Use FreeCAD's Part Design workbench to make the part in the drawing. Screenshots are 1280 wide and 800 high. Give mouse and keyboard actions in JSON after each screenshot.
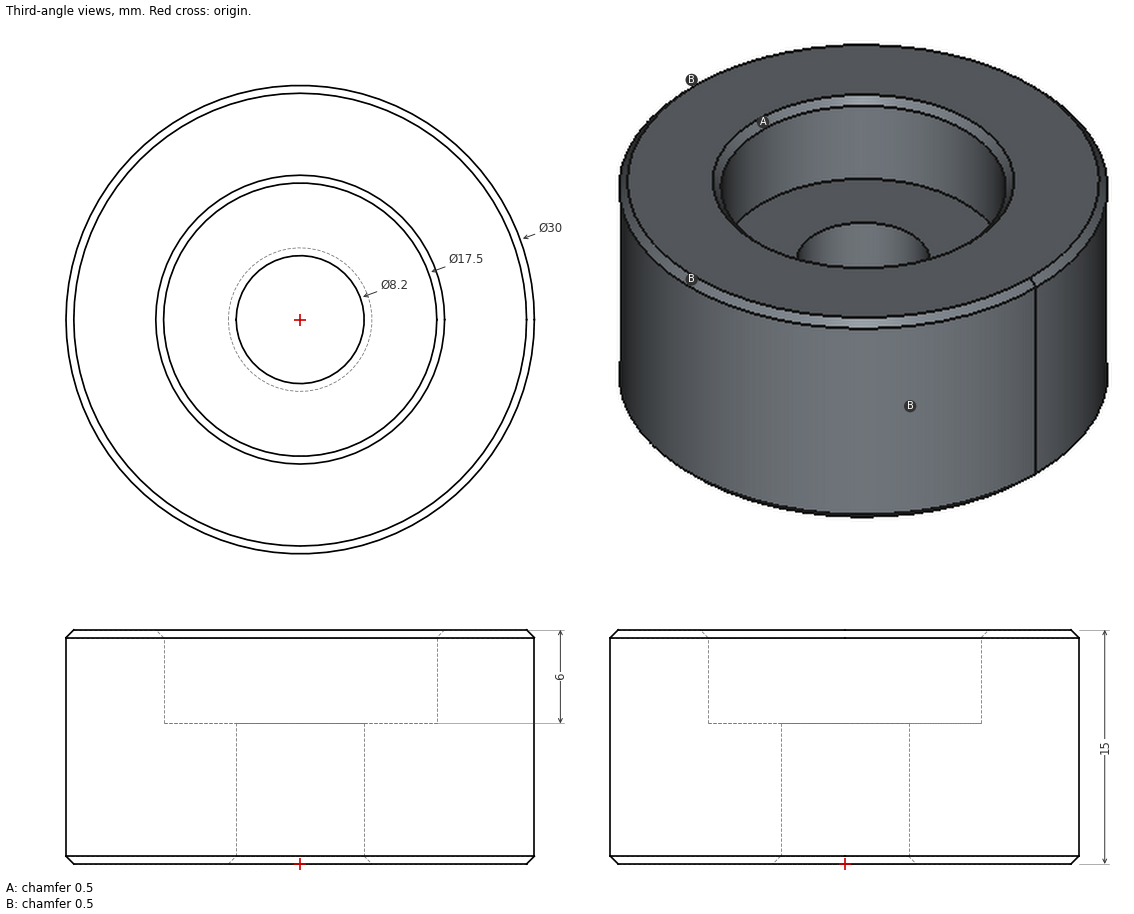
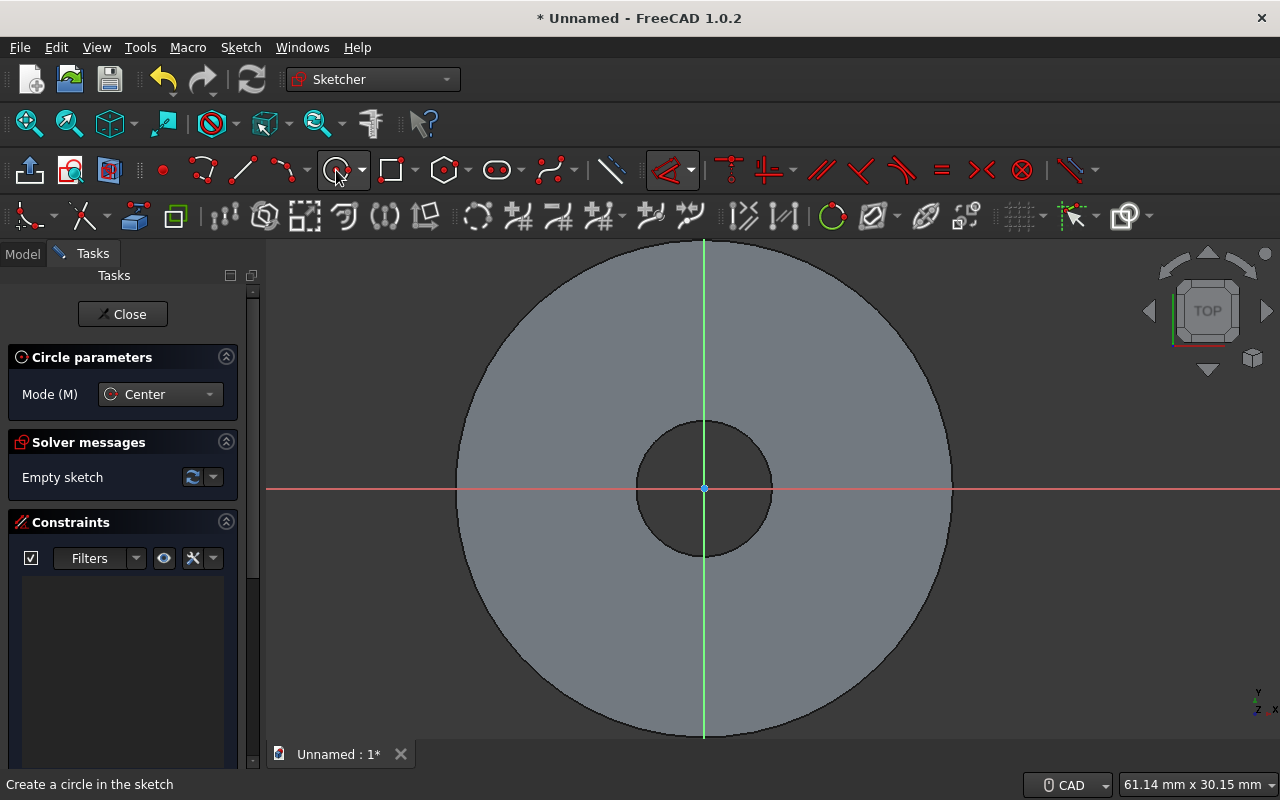
{"action": "left_click", "coordinate": [704, 489]}
{"action": "mouse_move", "coordinate": [807, 386]}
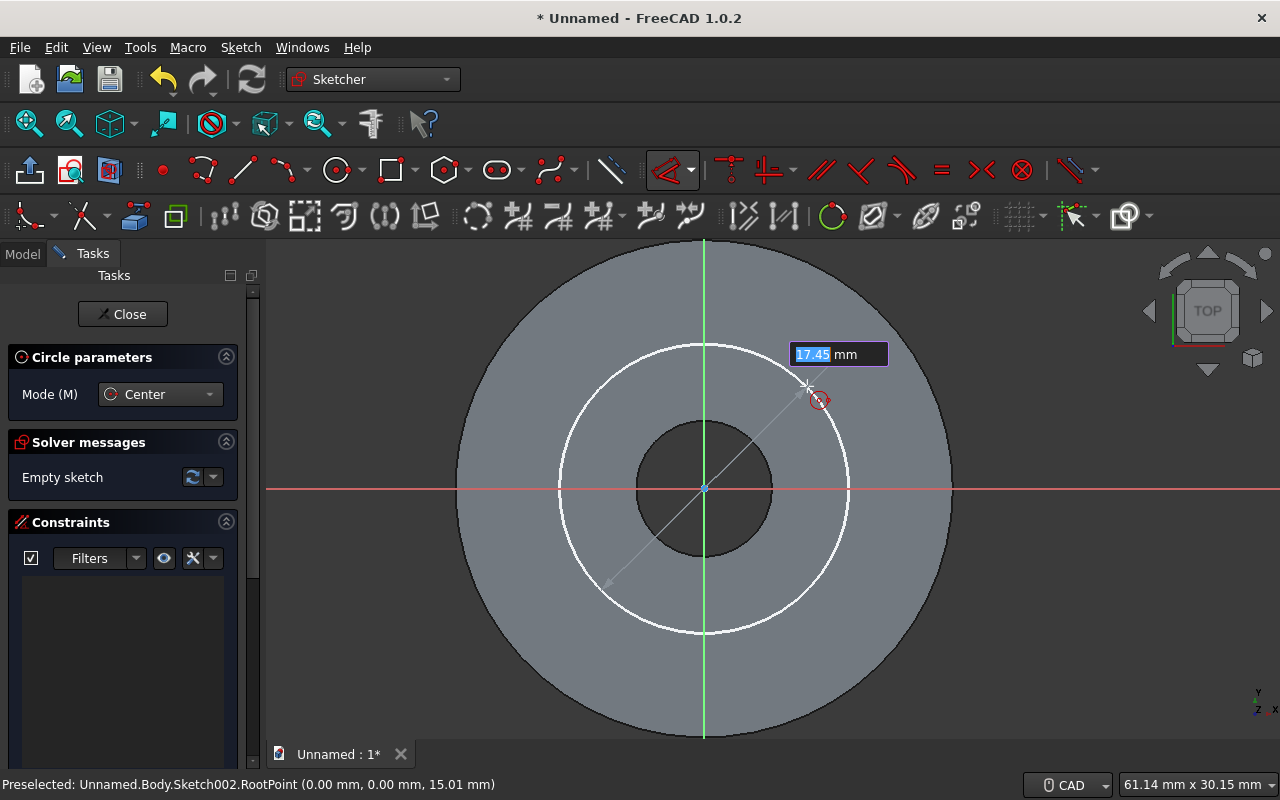
{"action": "type", "text": "17.5"}
{"action": "key", "text": "Return"}
{"action": "key", "text": "Escape"}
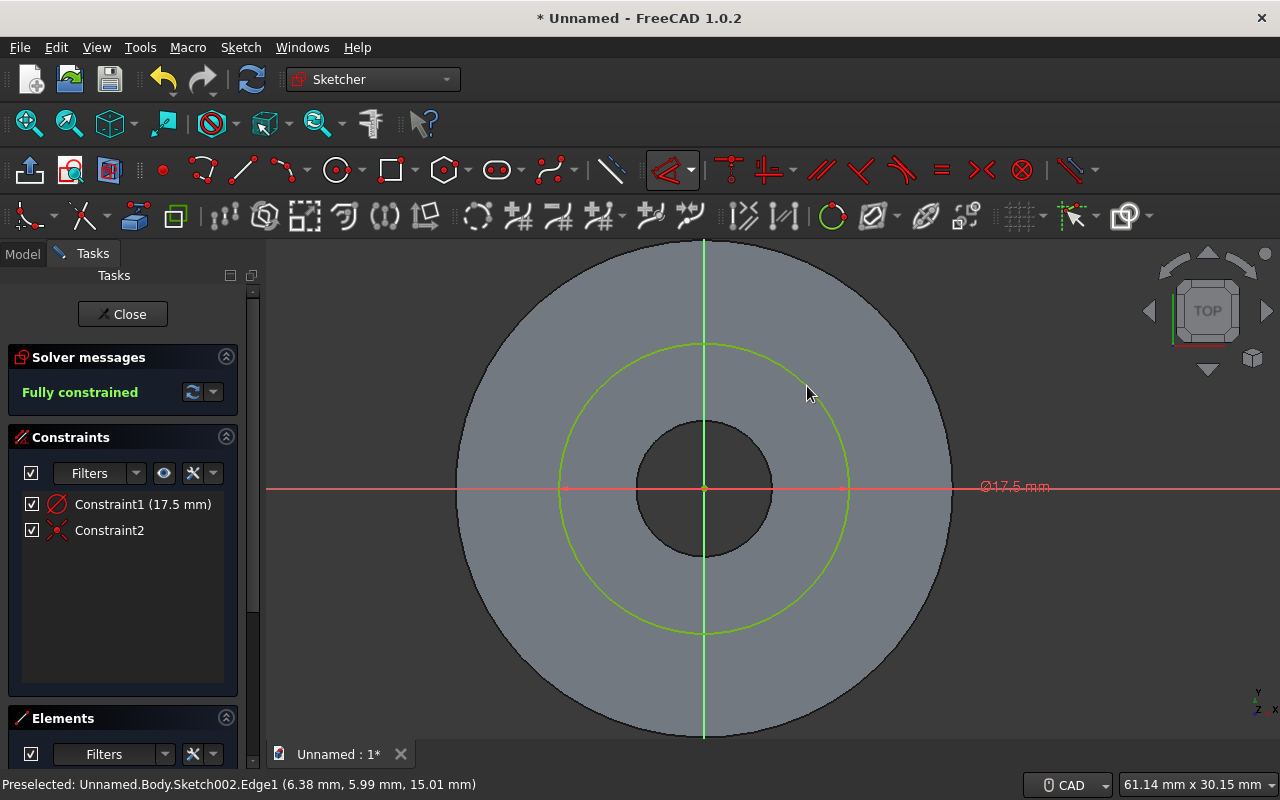
{"action": "left_click", "coordinate": [123, 314]}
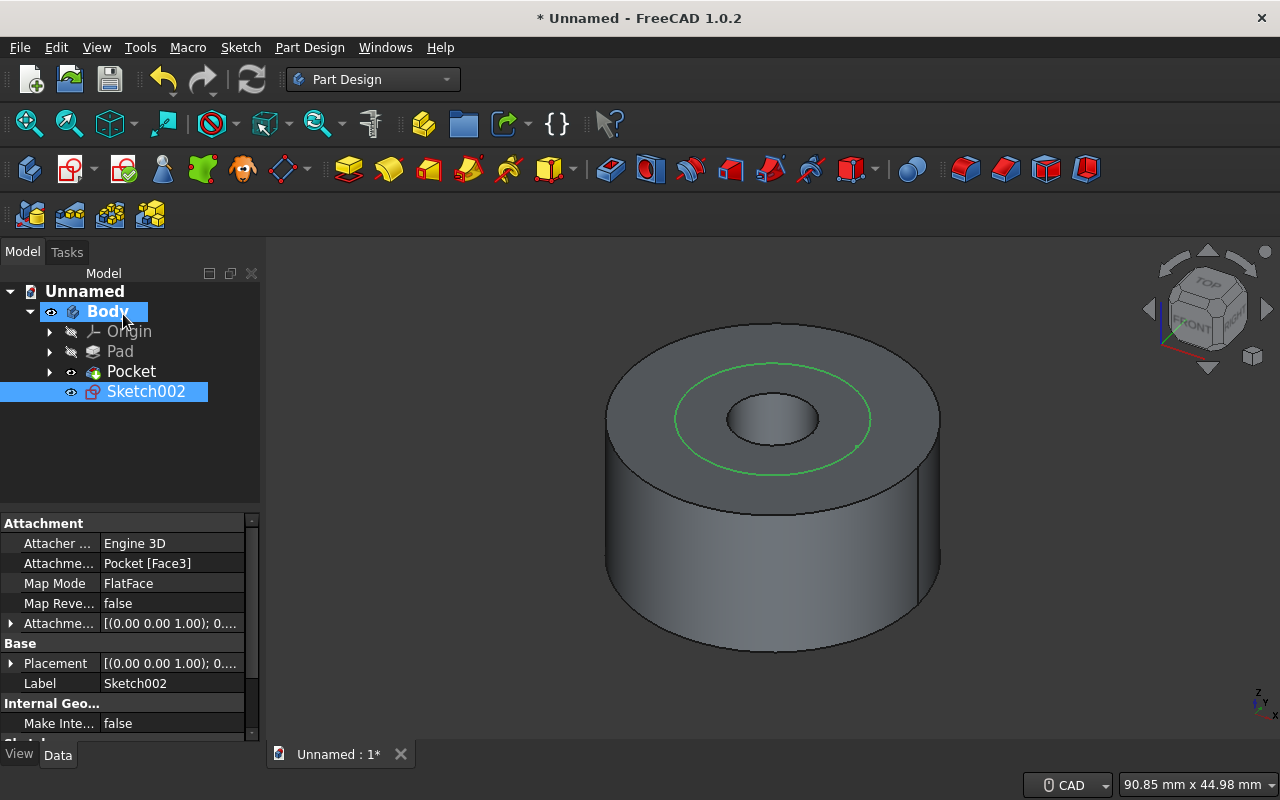
{"action": "left_click", "coordinate": [612, 170]}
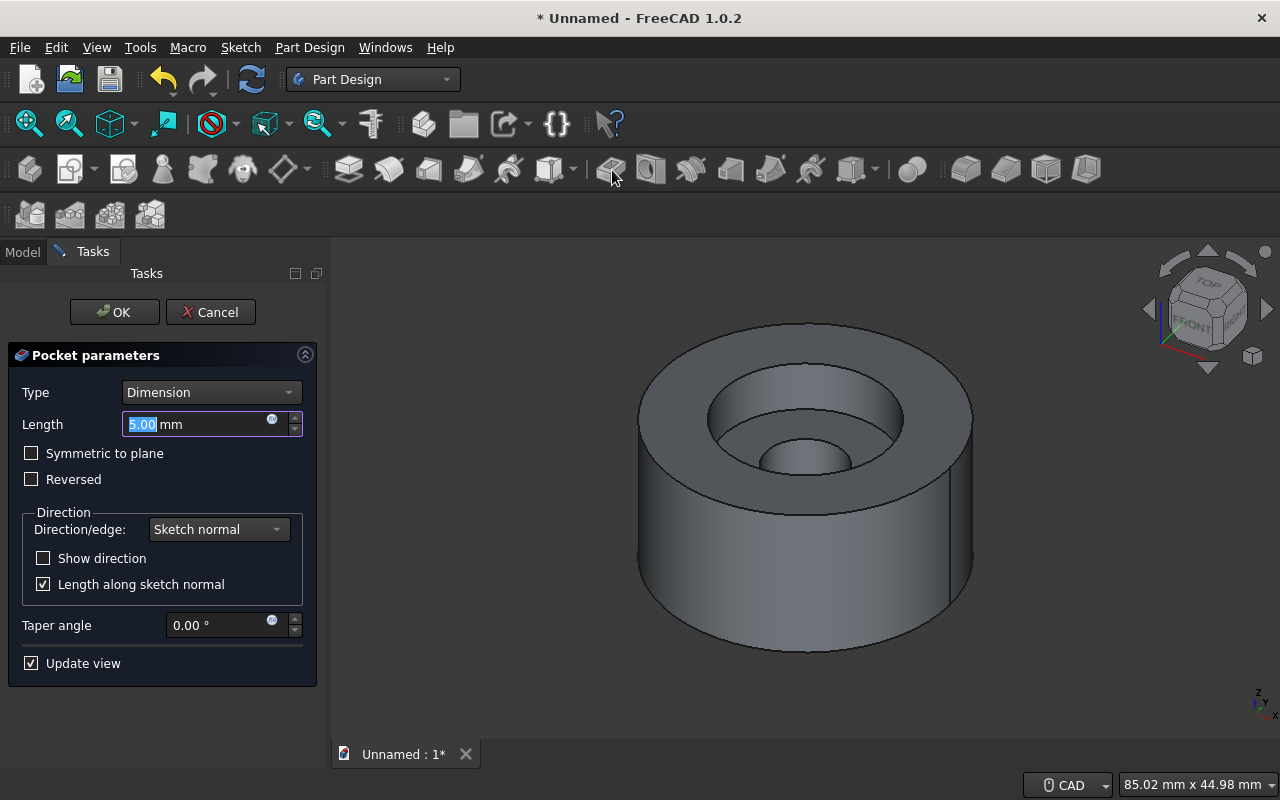
{"action": "type", "text": "6"}
{"action": "key", "text": "Tab"}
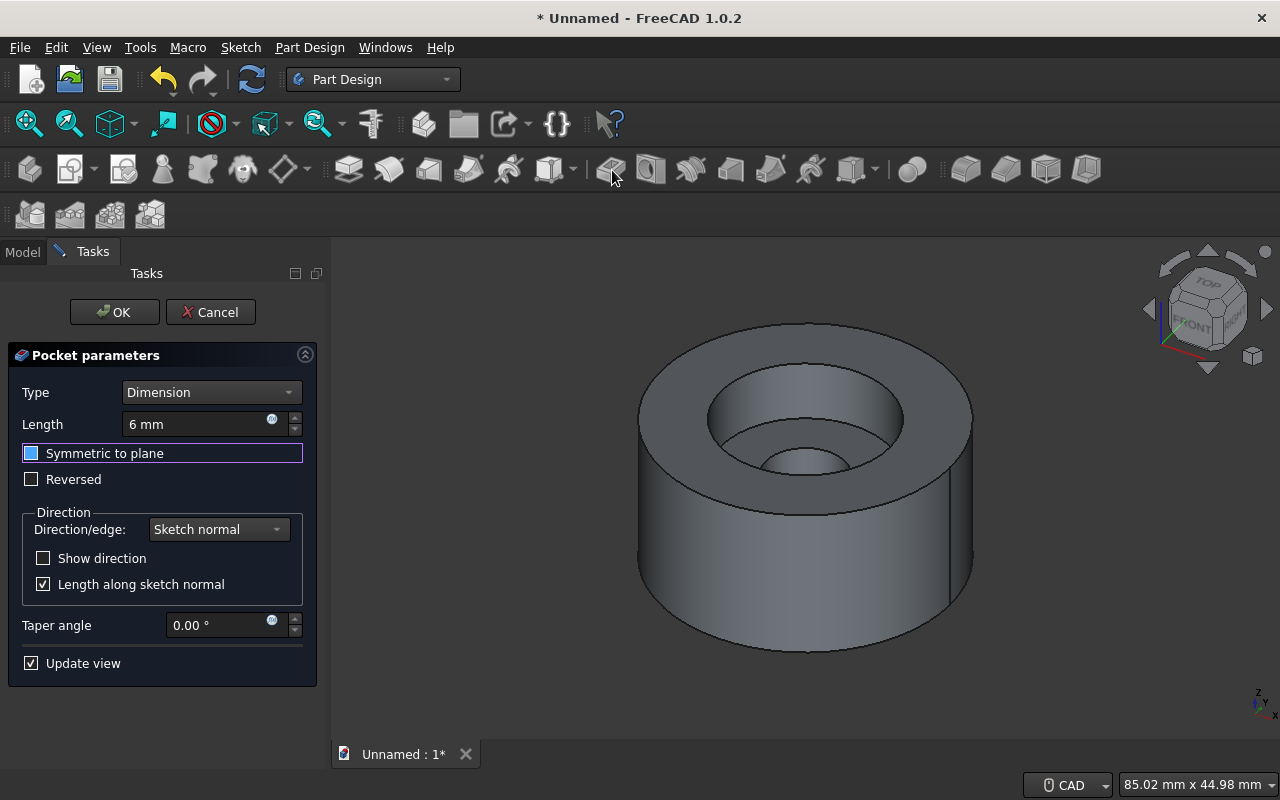
{"action": "left_click", "coordinate": [115, 312]}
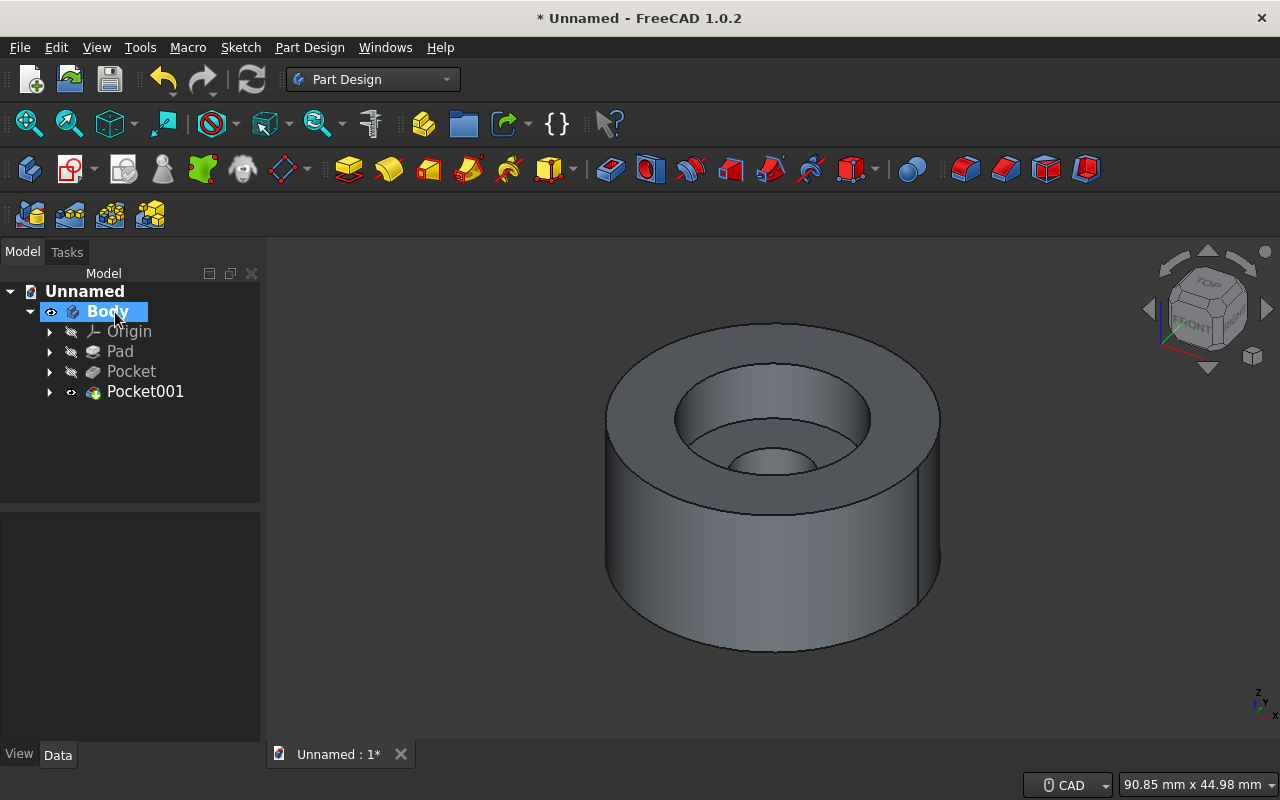
{"action": "left_click", "coordinate": [688, 390]}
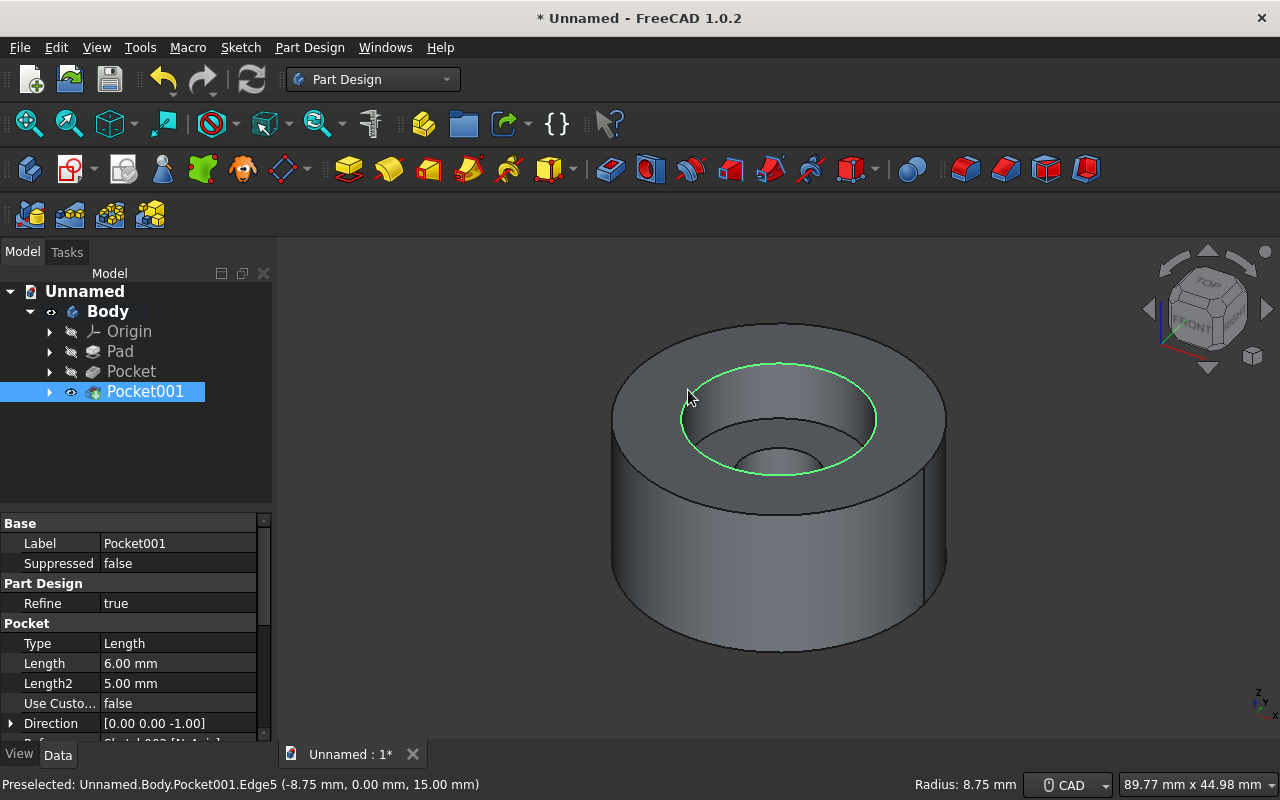
{"action": "left_click", "coordinate": [1006, 170]}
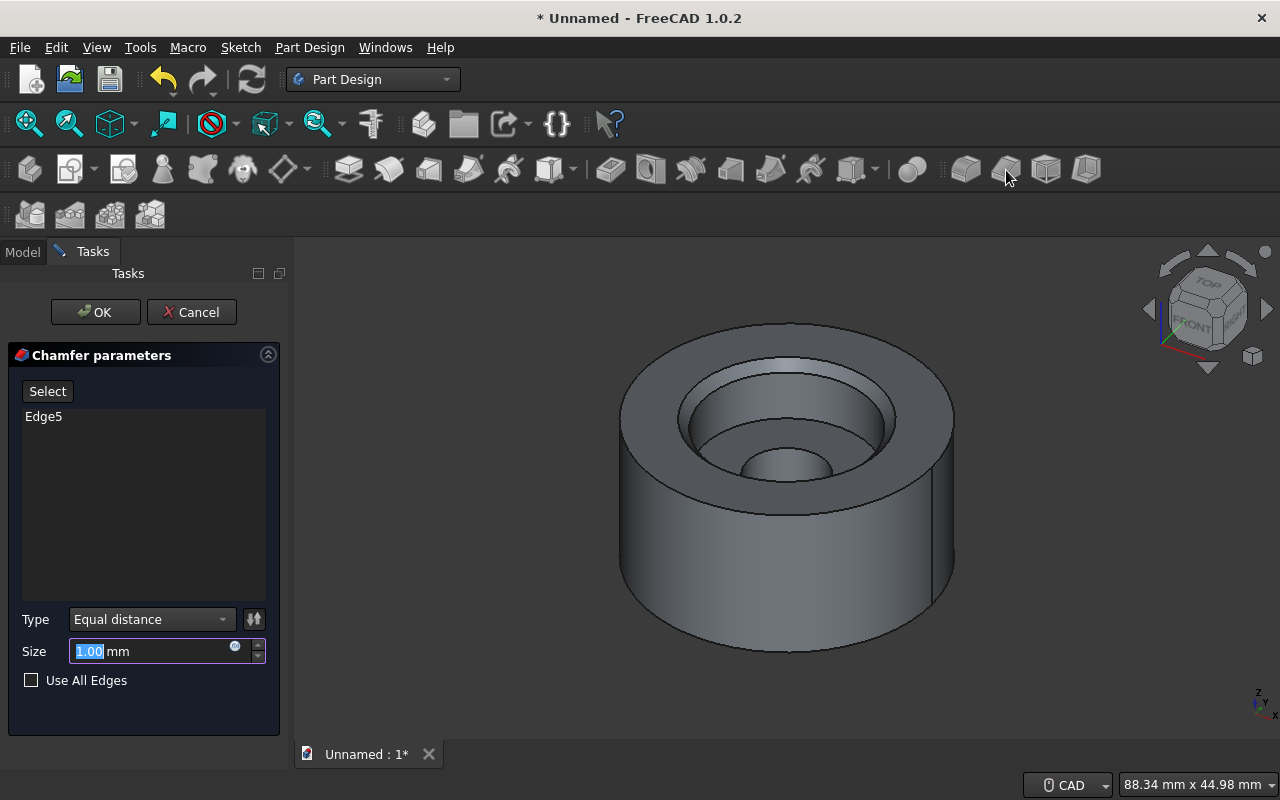
{"action": "type", "text": "0.5"}
{"action": "key", "text": "Tab"}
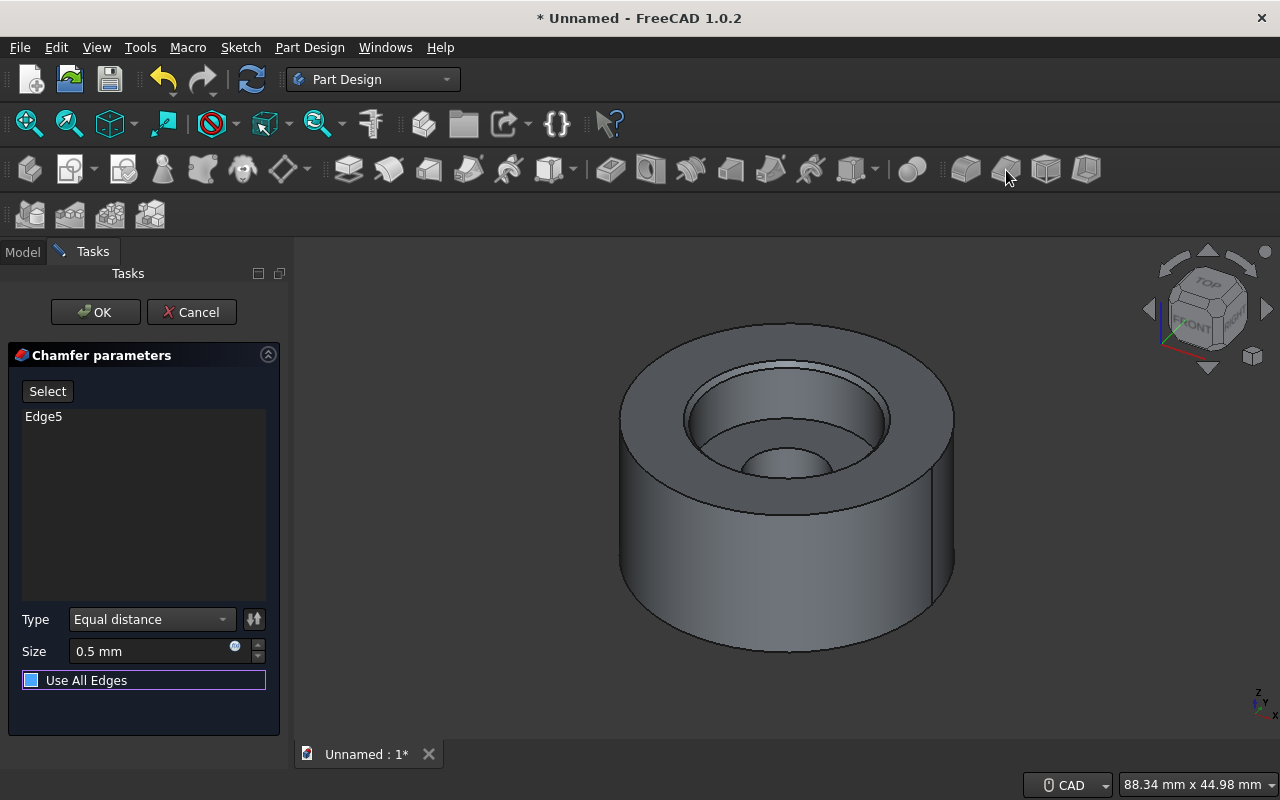
{"action": "left_click", "coordinate": [96, 312]}